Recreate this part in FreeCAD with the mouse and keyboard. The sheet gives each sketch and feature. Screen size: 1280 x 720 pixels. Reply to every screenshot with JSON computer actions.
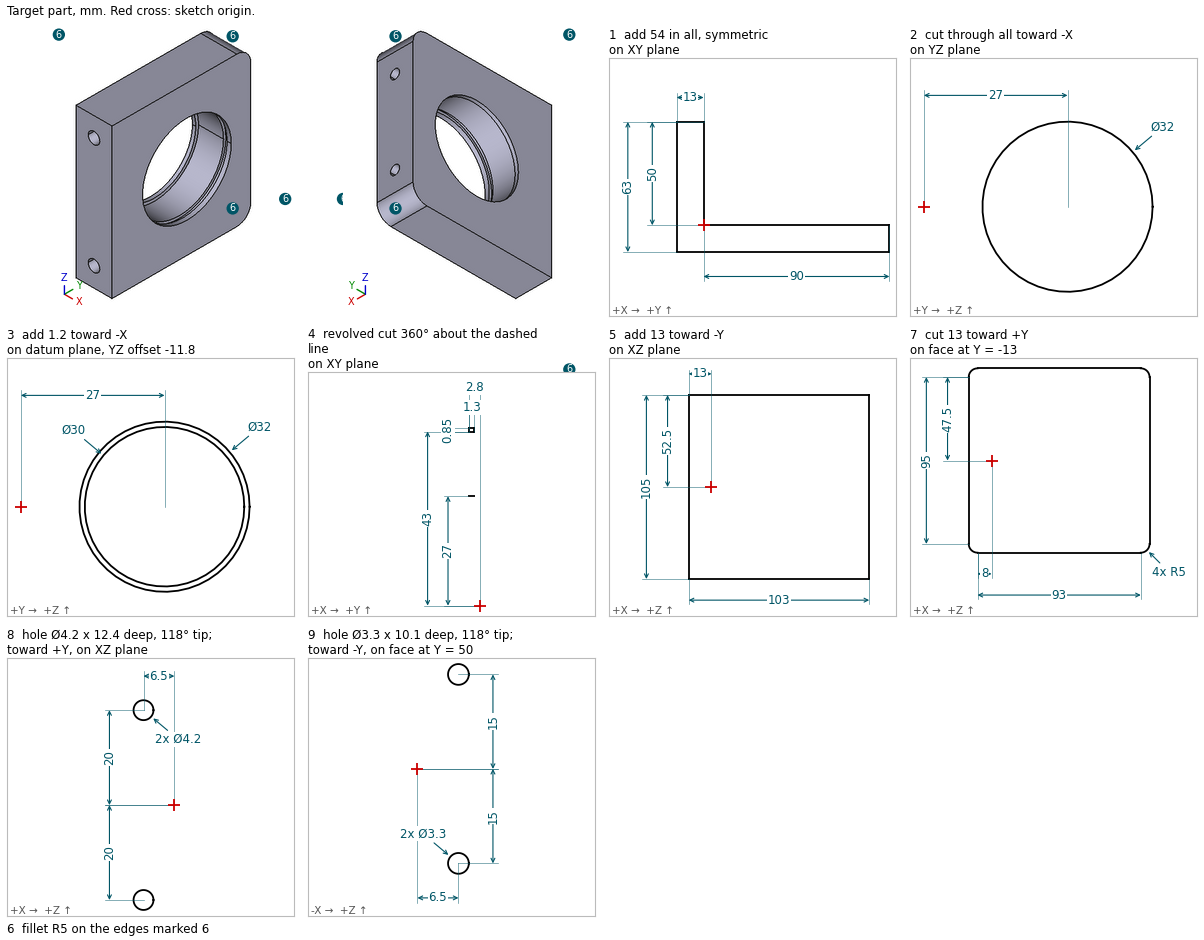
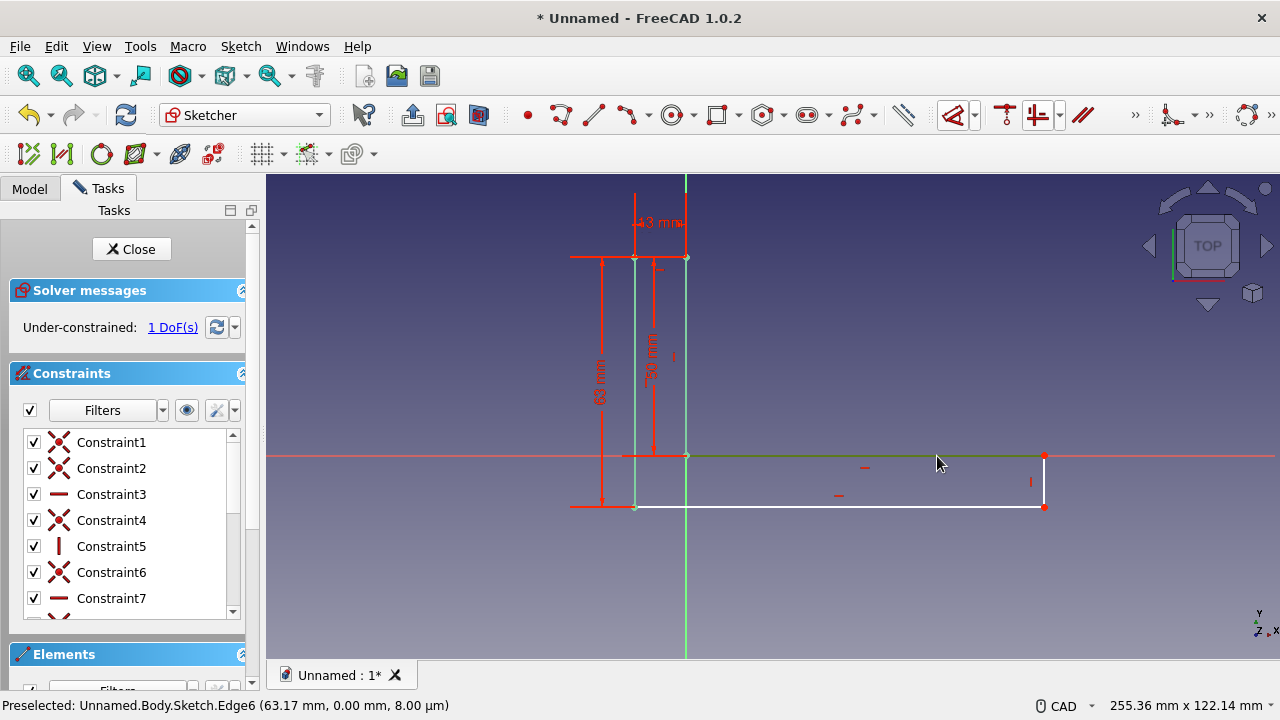
{"action": "left_click", "coordinate": [974, 116]}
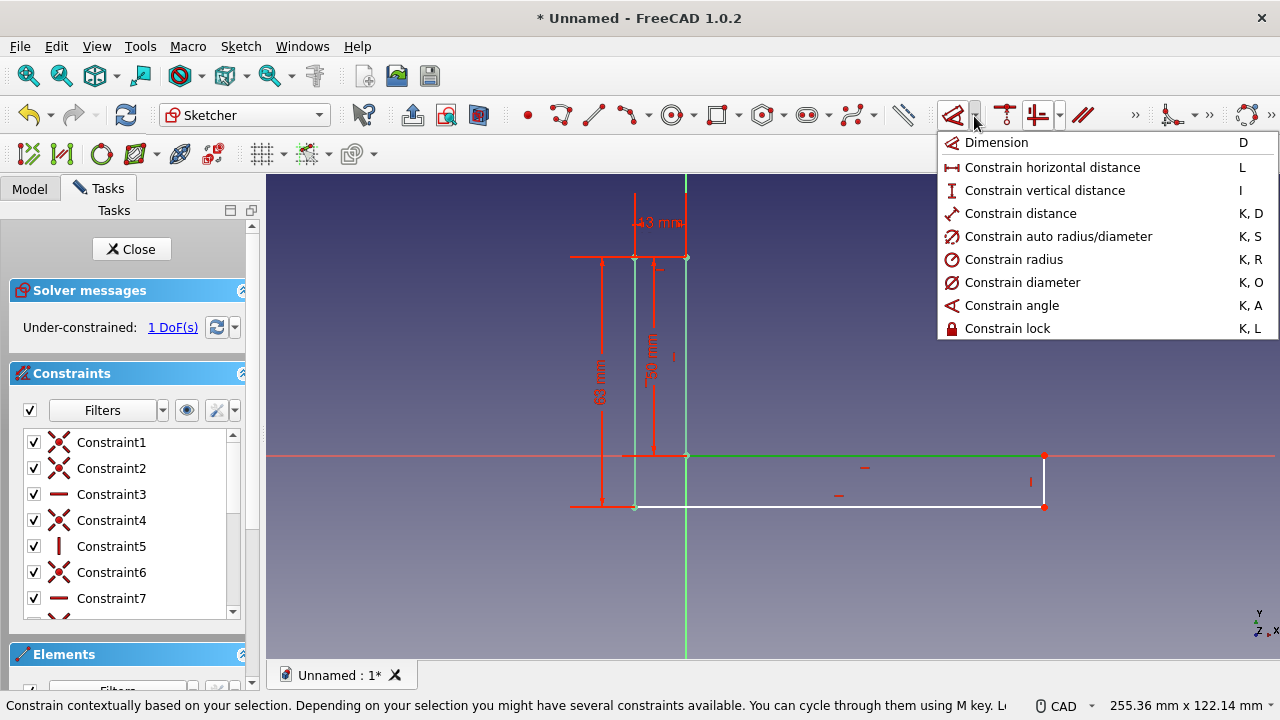
{"action": "left_click", "coordinate": [1108, 168]}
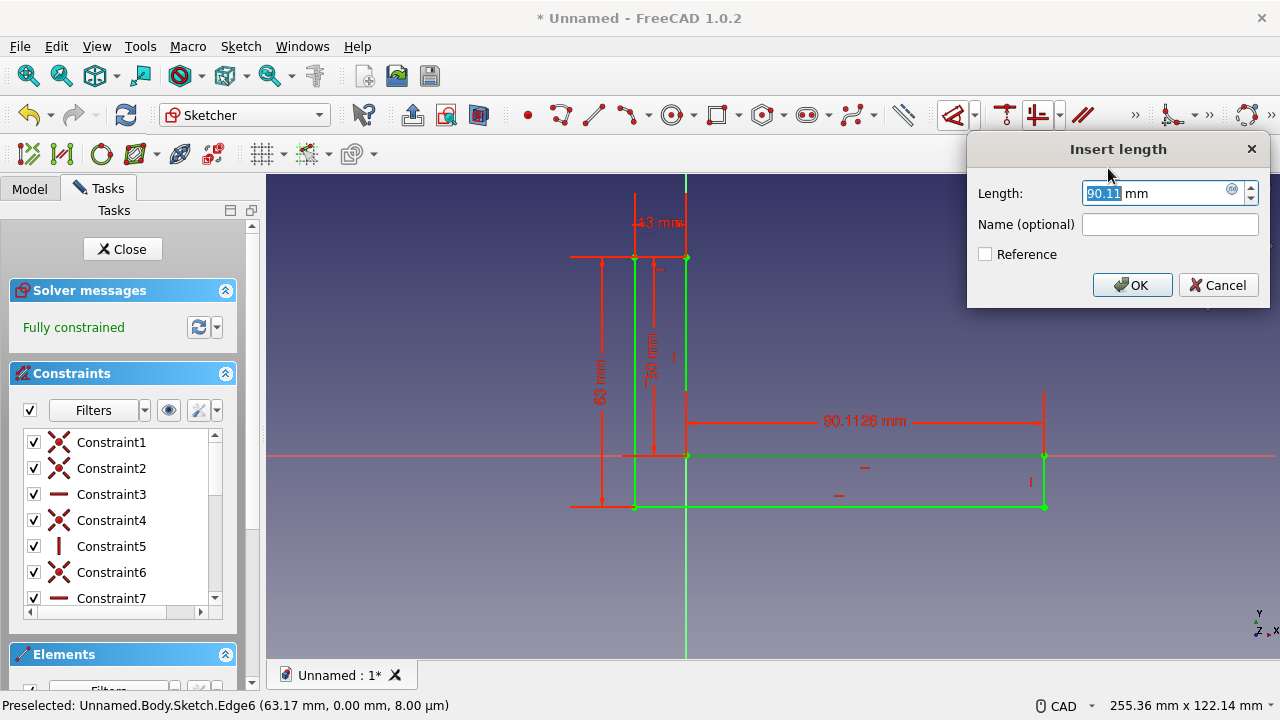
{"action": "type", "text": "90"}
{"action": "key", "text": "Return"}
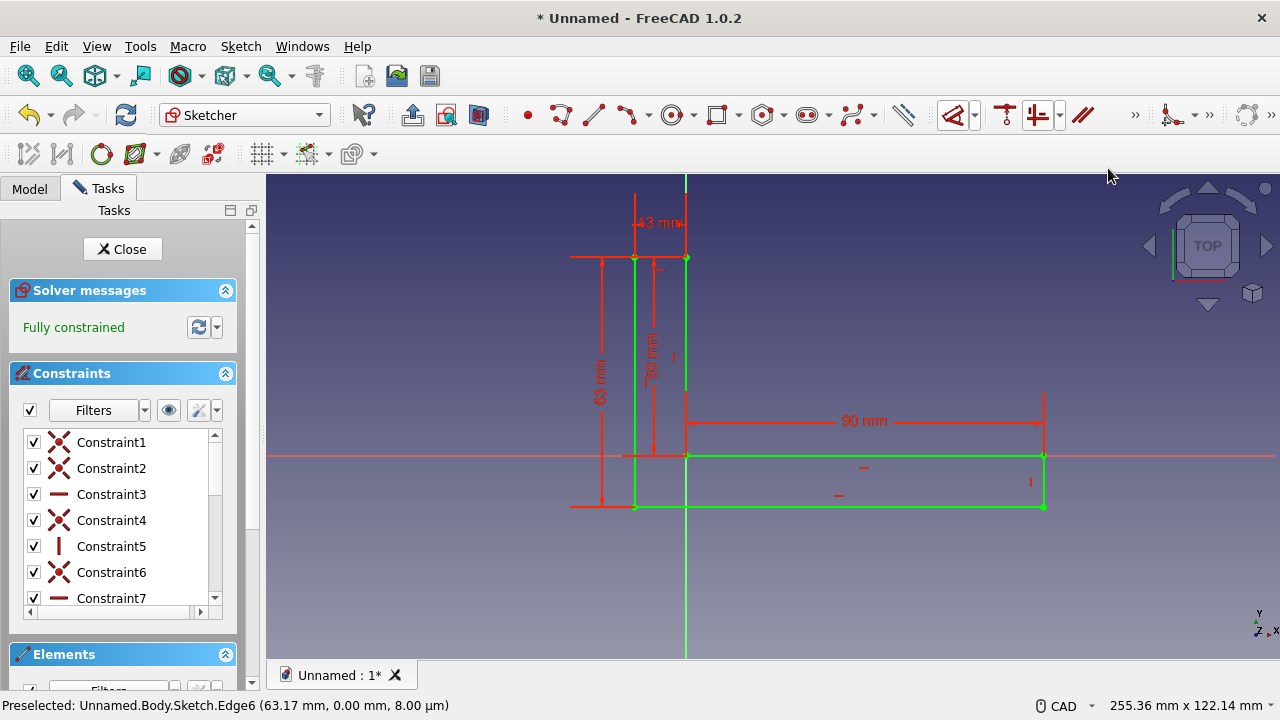
{"action": "left_click", "coordinate": [123, 249]}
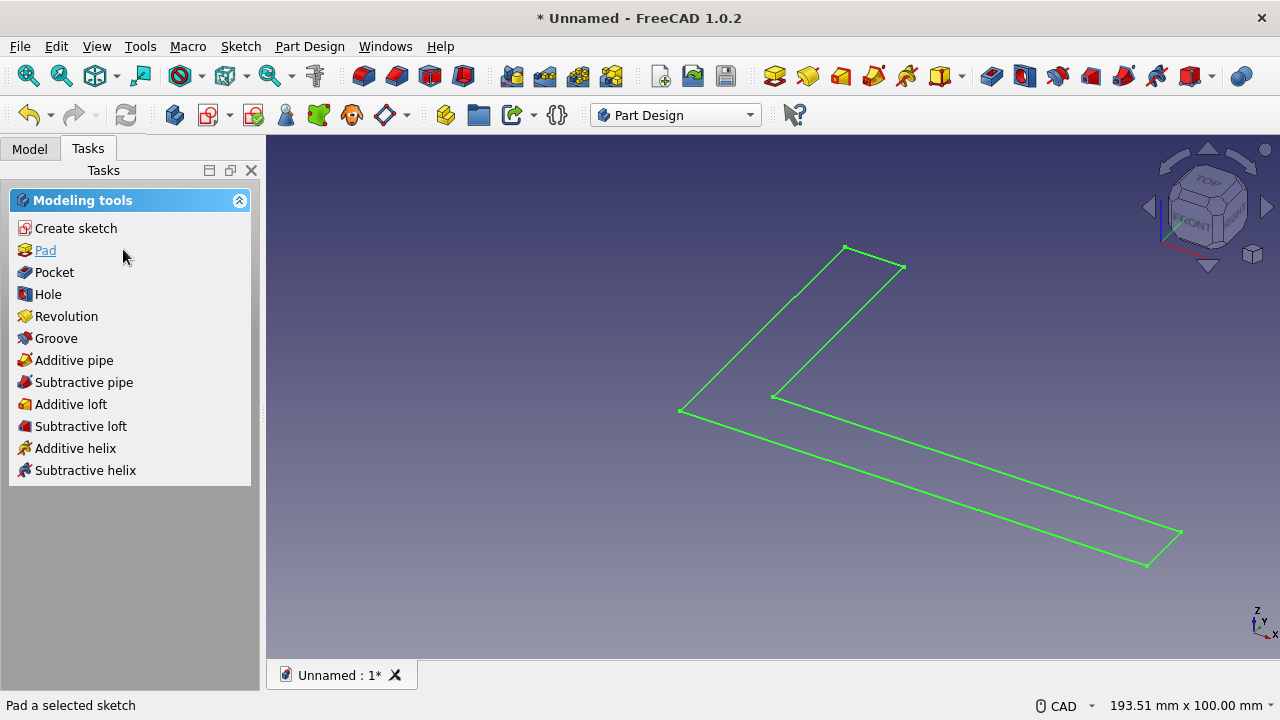
{"action": "left_click", "coordinate": [775, 76]}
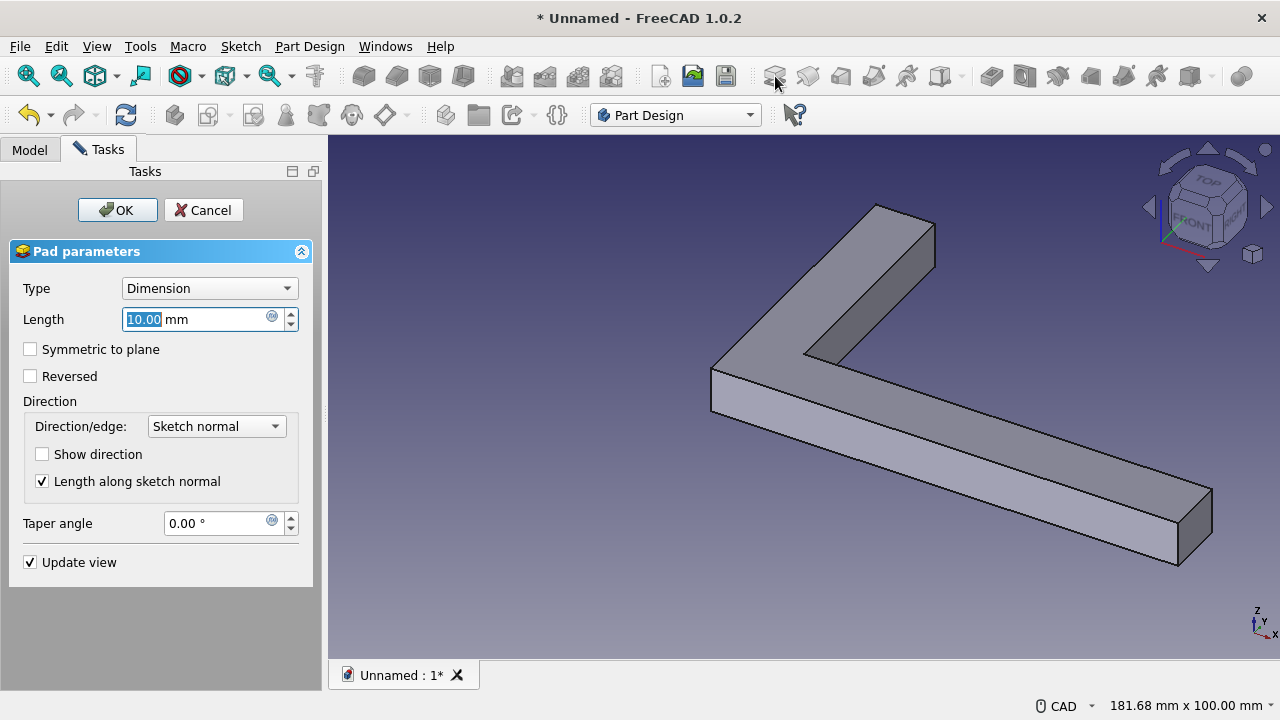
{"action": "type", "text": "54"}
{"action": "key", "text": "Tab"}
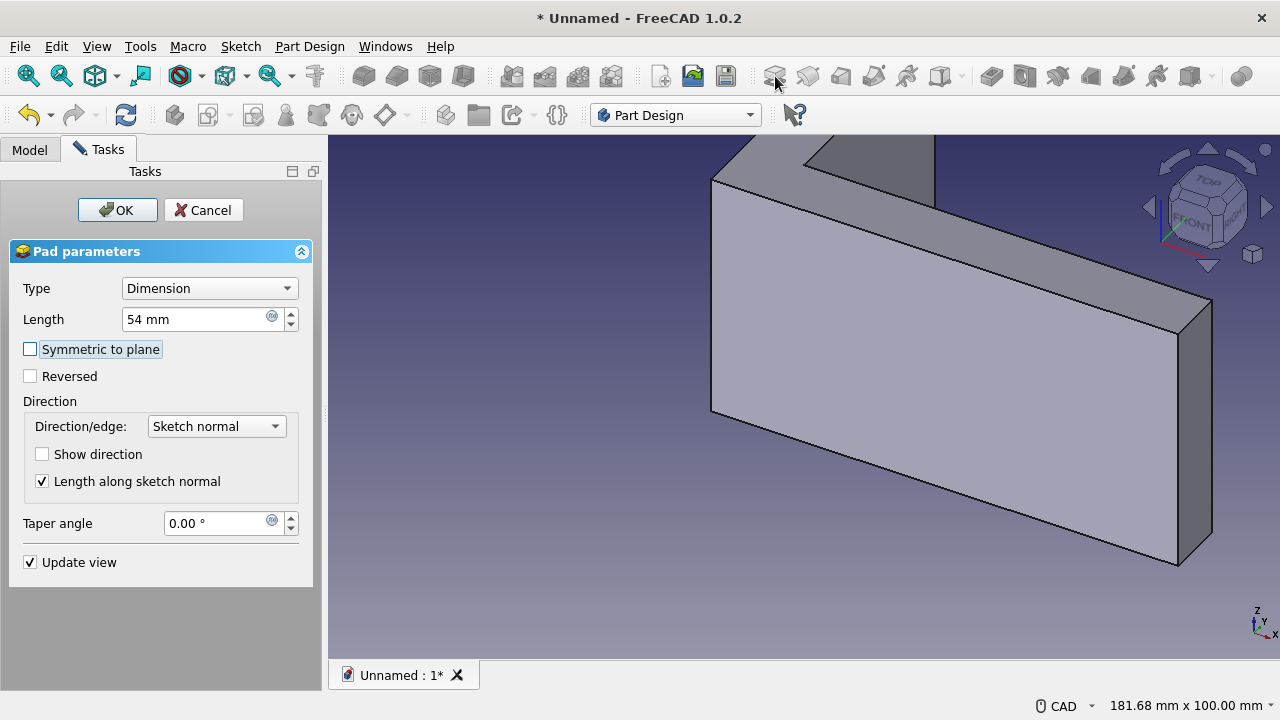
{"action": "left_click", "coordinate": [31, 349]}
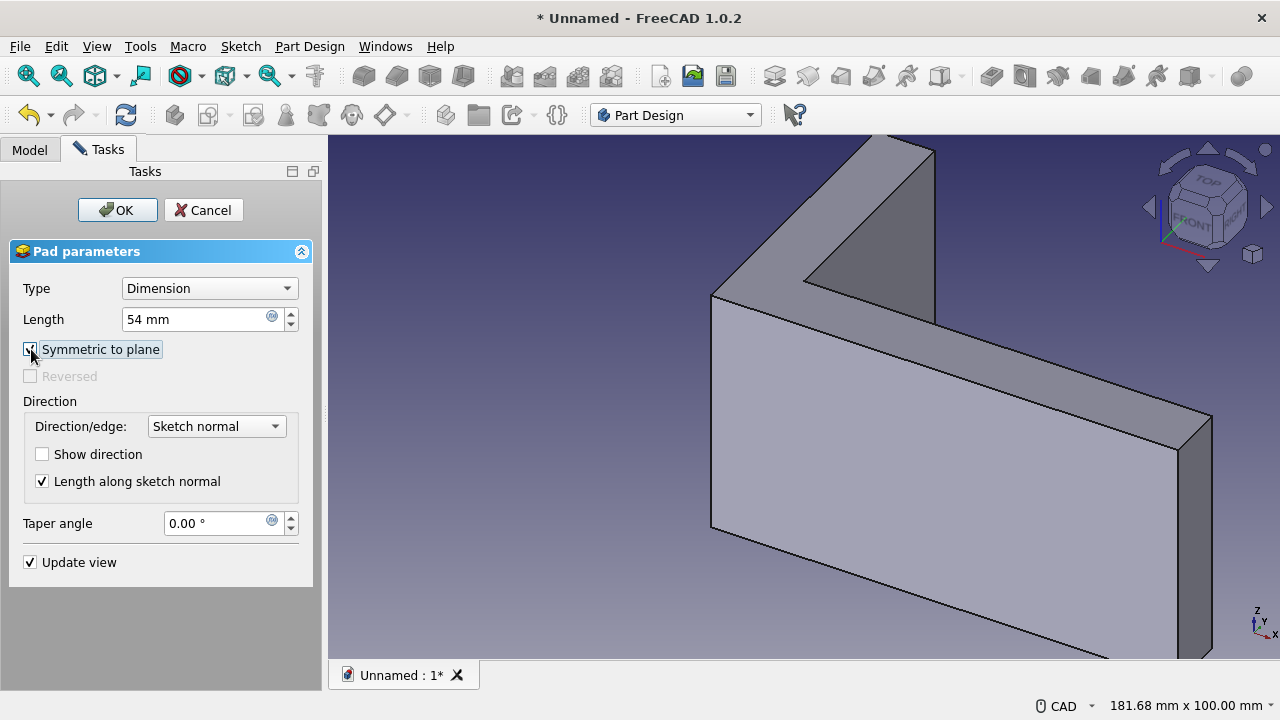
{"action": "left_click", "coordinate": [118, 210]}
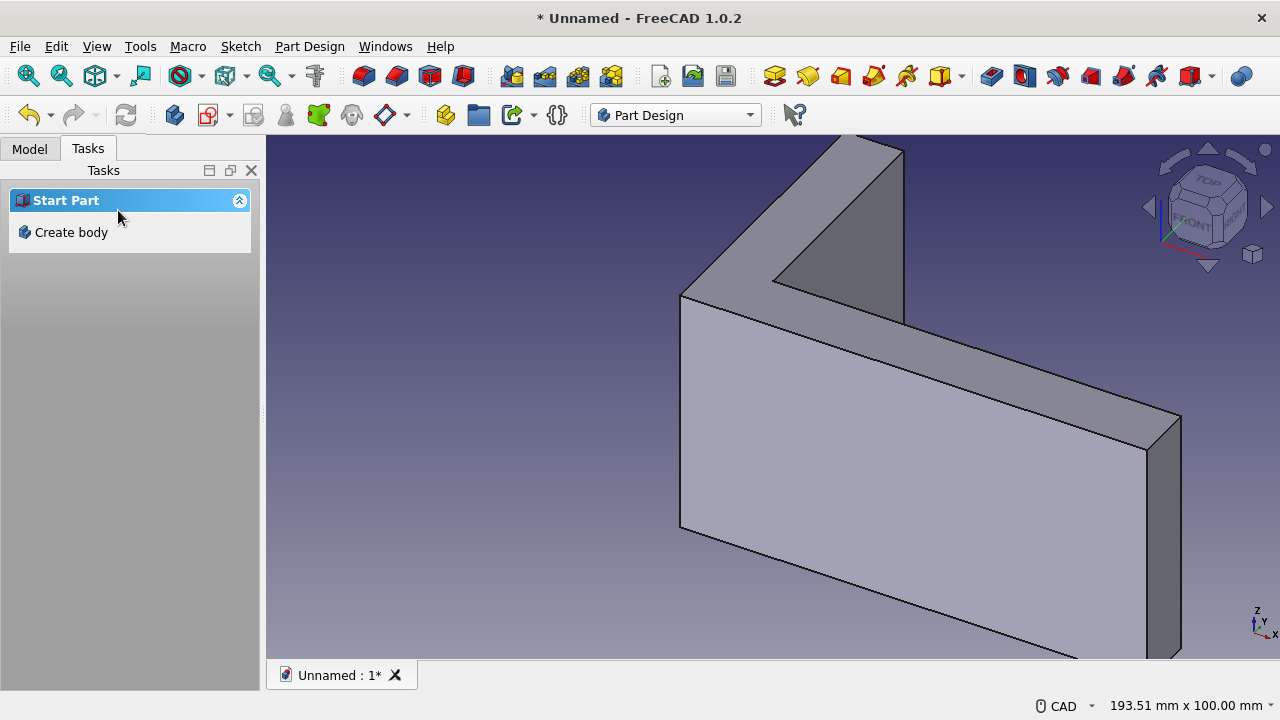
{"action": "left_click", "coordinate": [29, 76]}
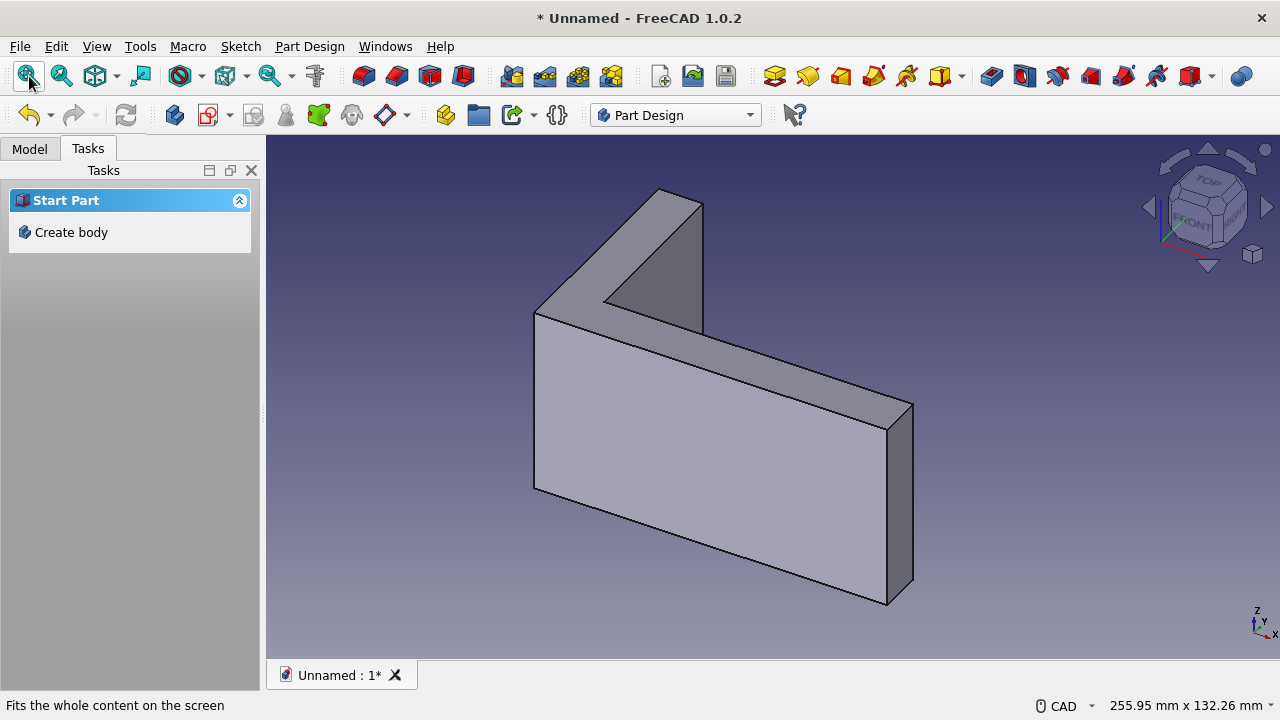
{"action": "left_click", "coordinate": [208, 116]}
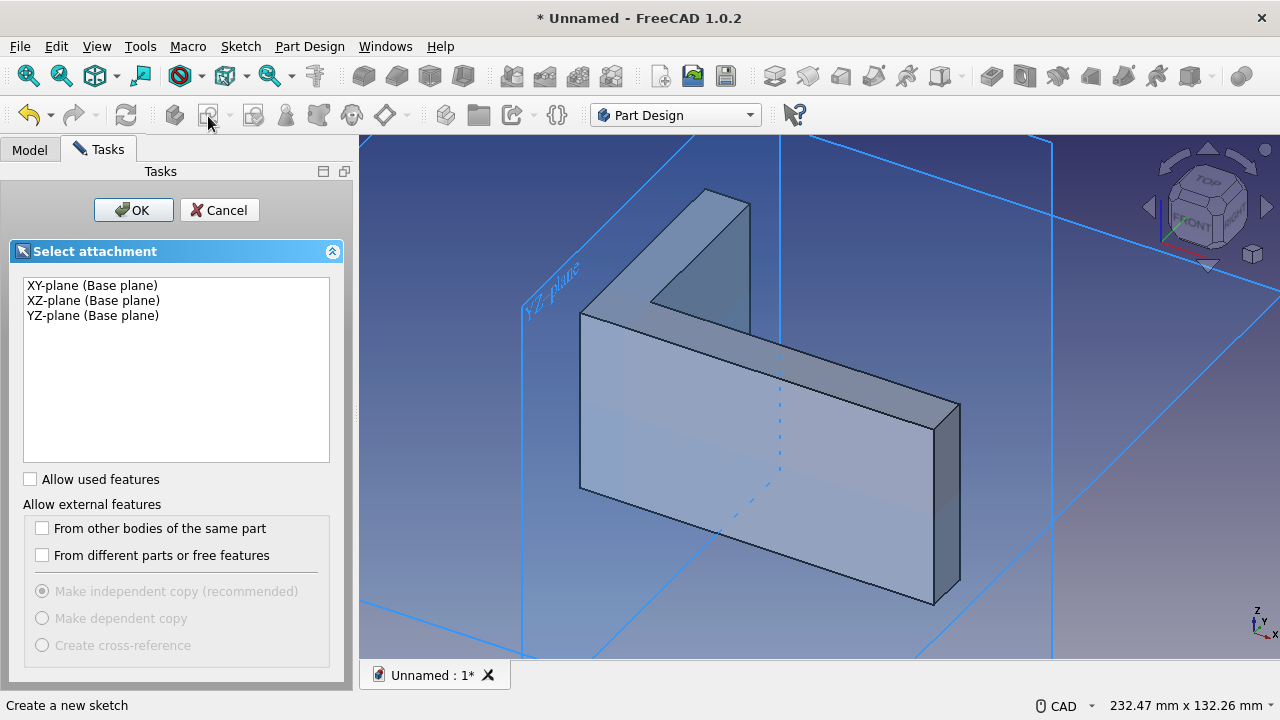
{"action": "left_click", "coordinate": [84, 316]}